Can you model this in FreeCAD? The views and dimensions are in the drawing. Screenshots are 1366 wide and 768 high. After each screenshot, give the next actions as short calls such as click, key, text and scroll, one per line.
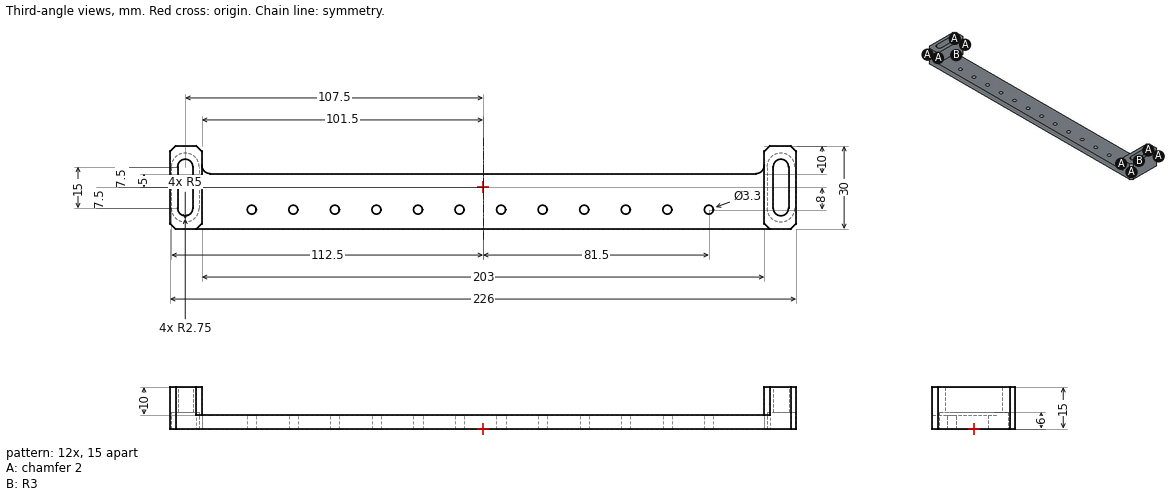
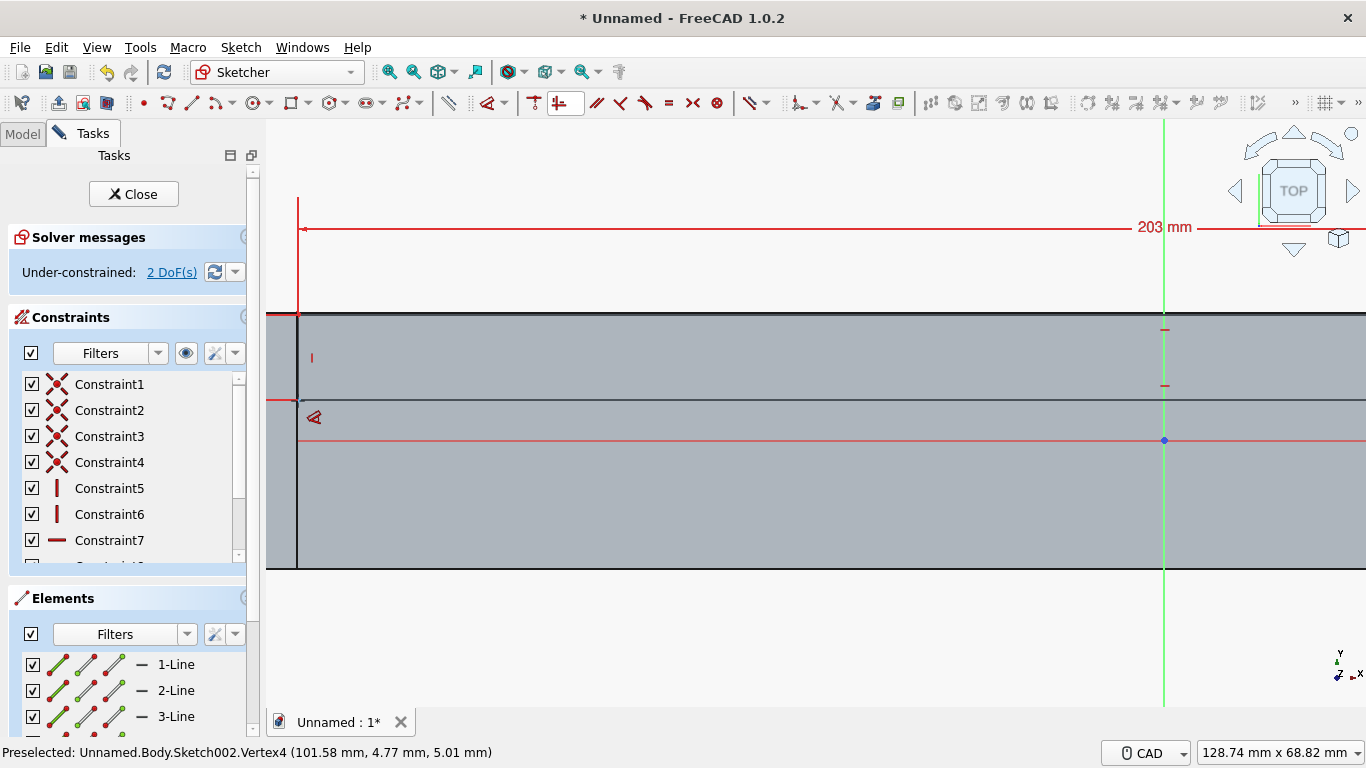
click(298, 400)
click(1198, 420)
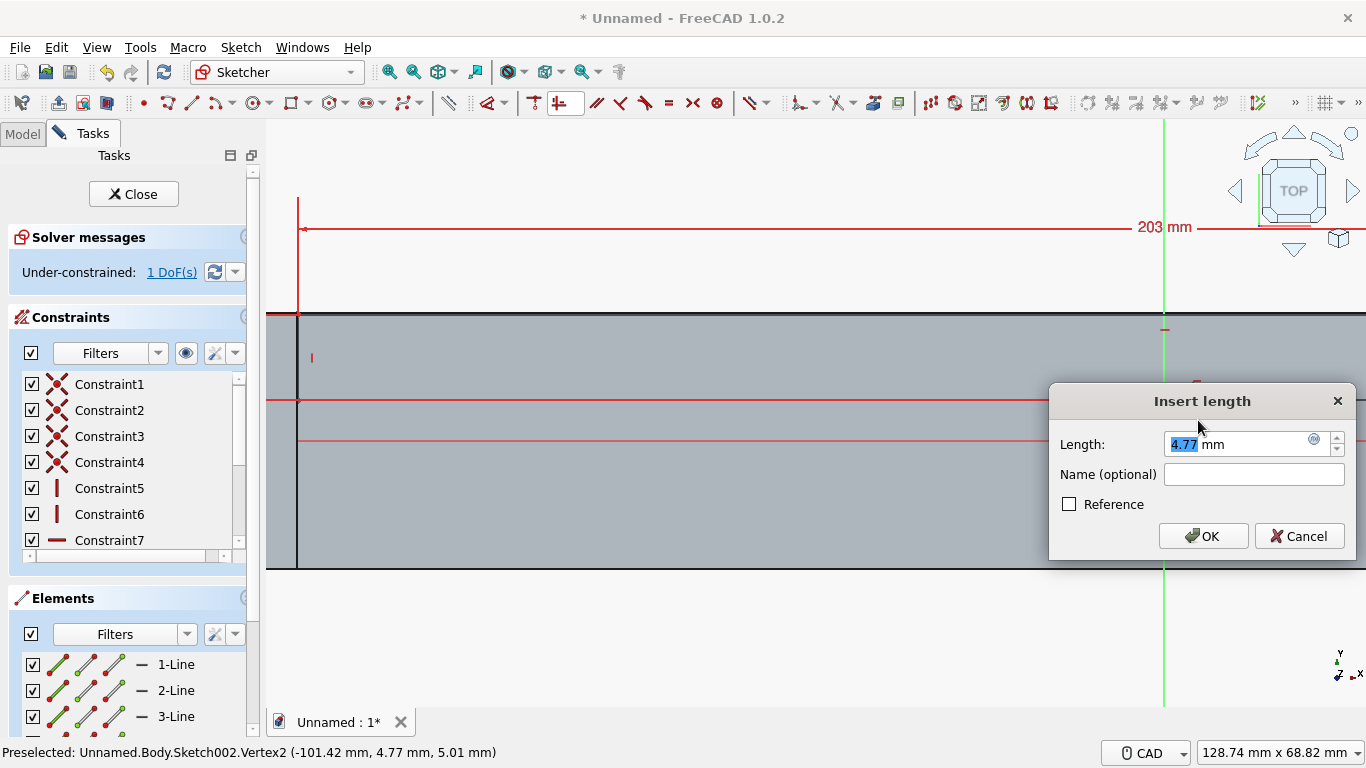
text(5)
key(Return)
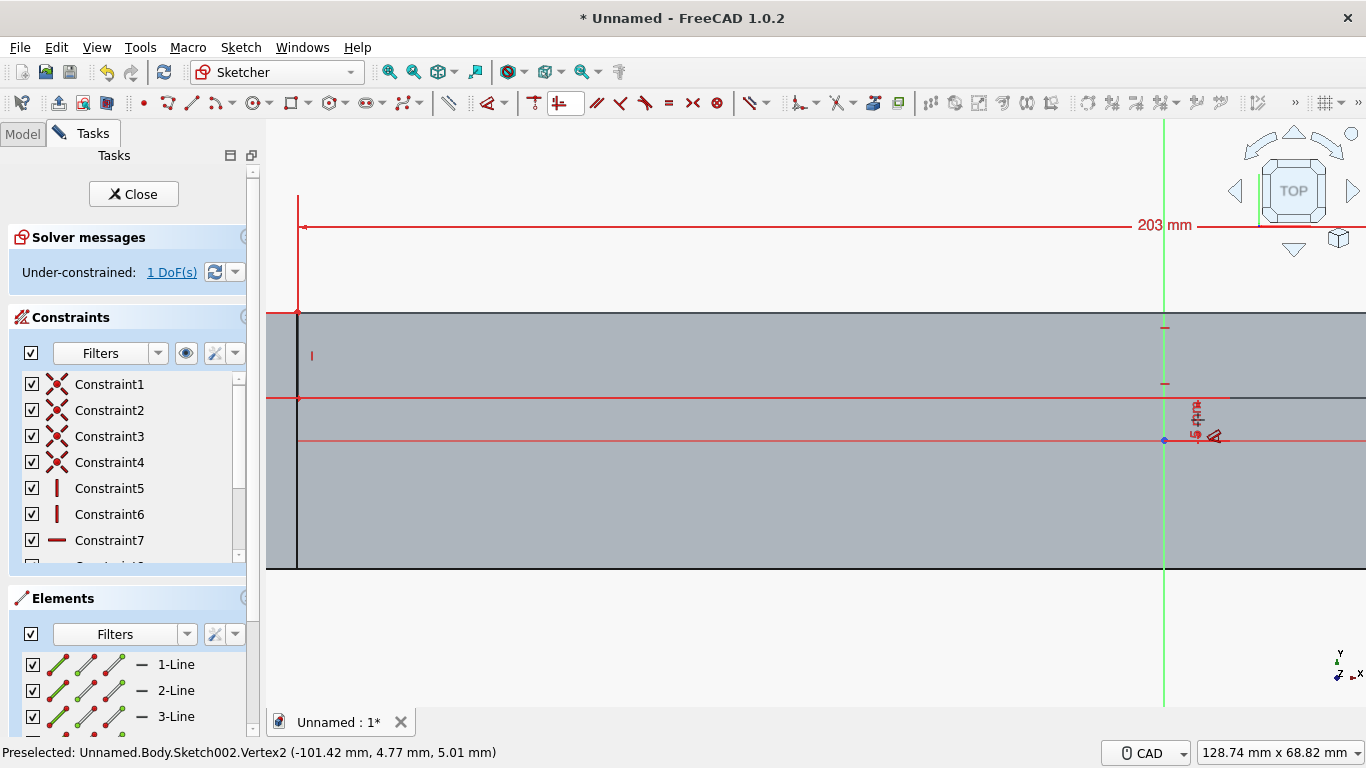
click(298, 313)
click(731, 475)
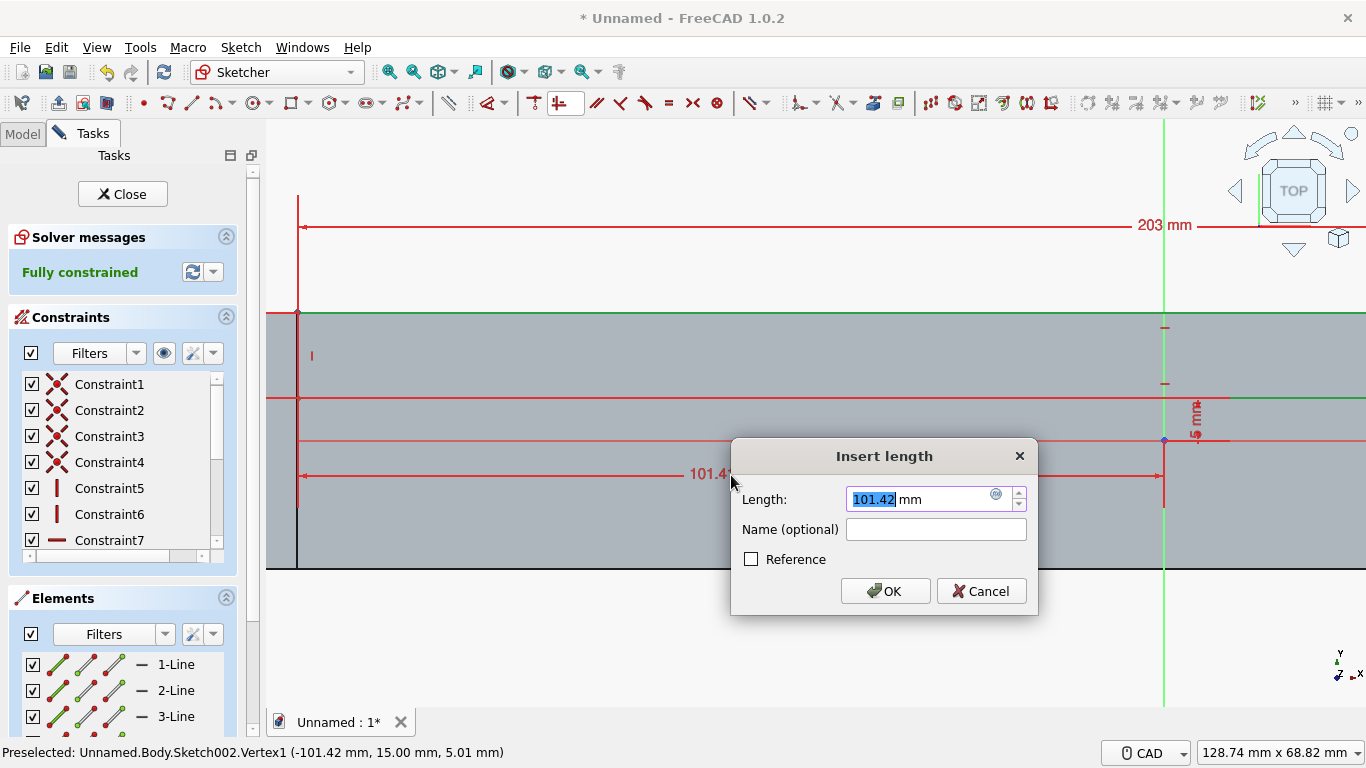
text(101.5)
key(Return)
key(Escape)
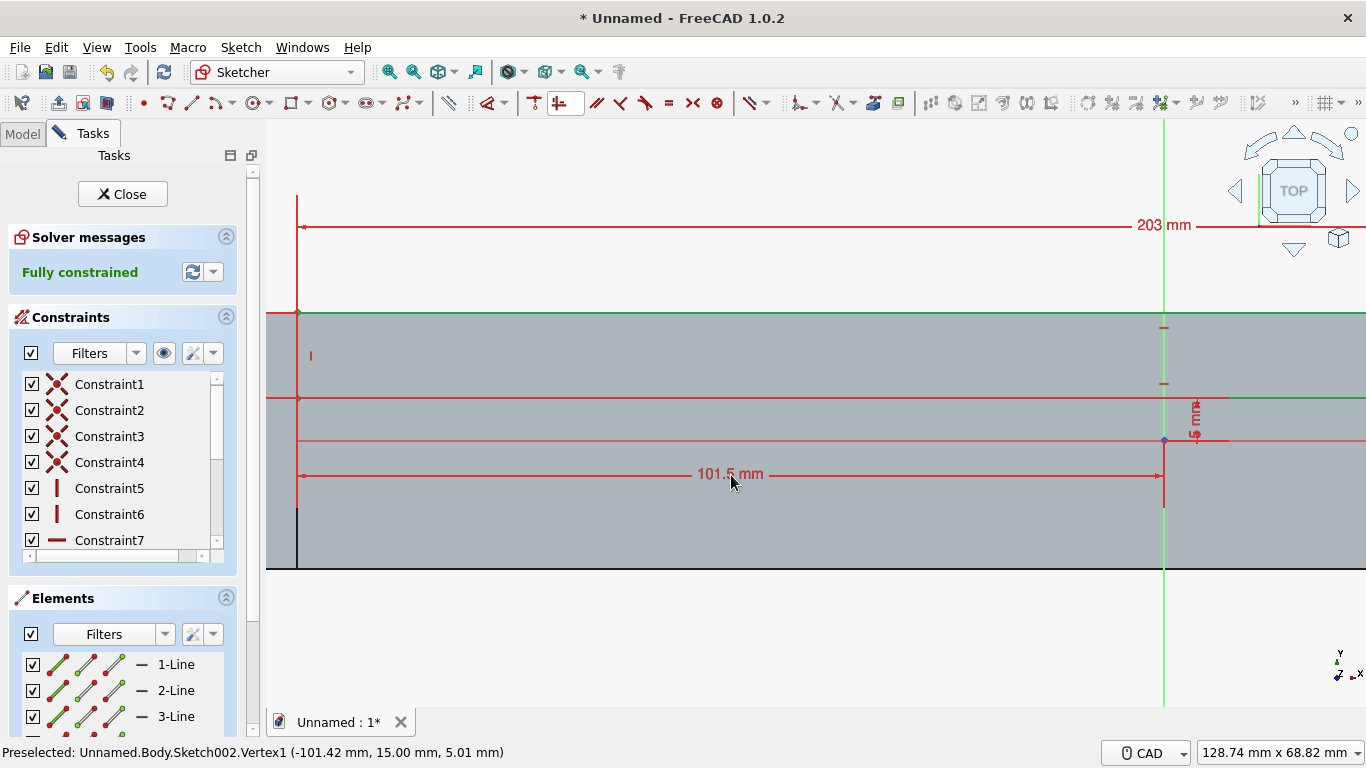
click(123, 194)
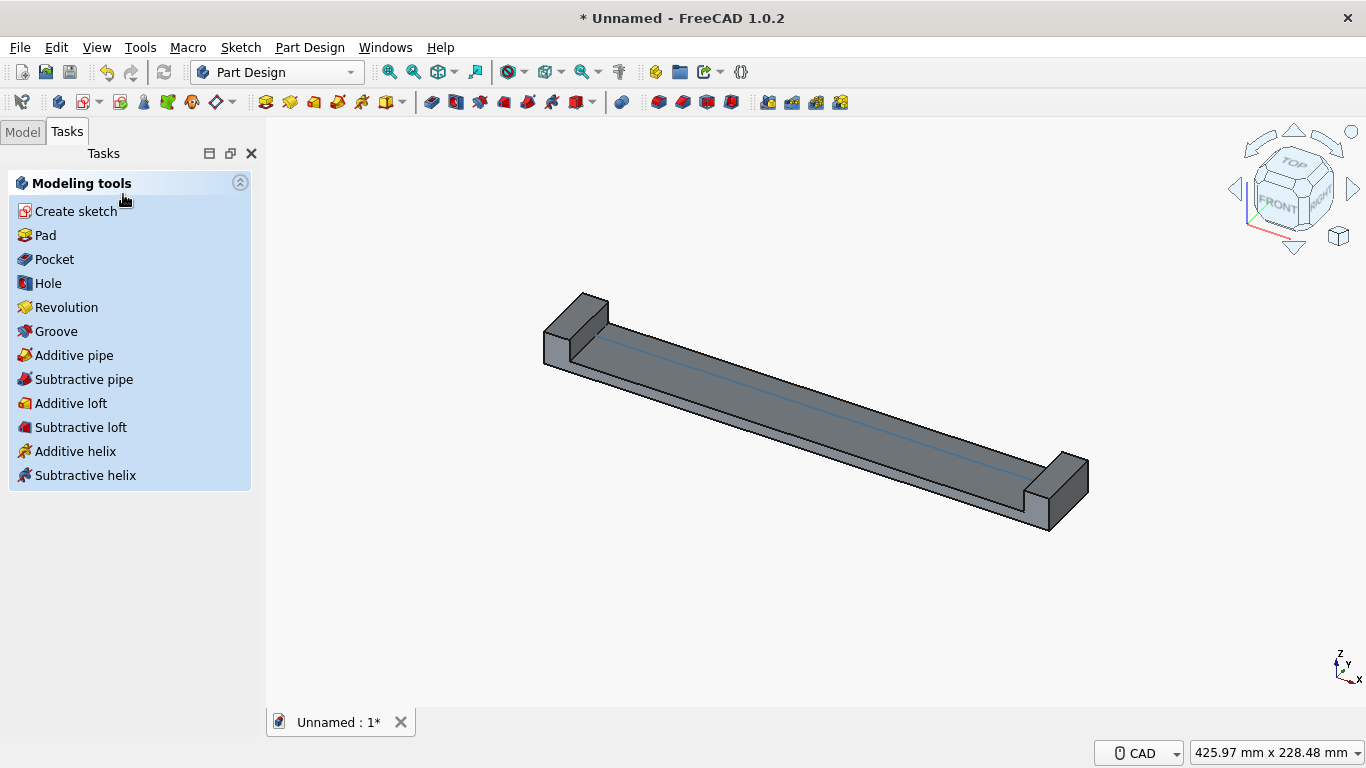
click(432, 102)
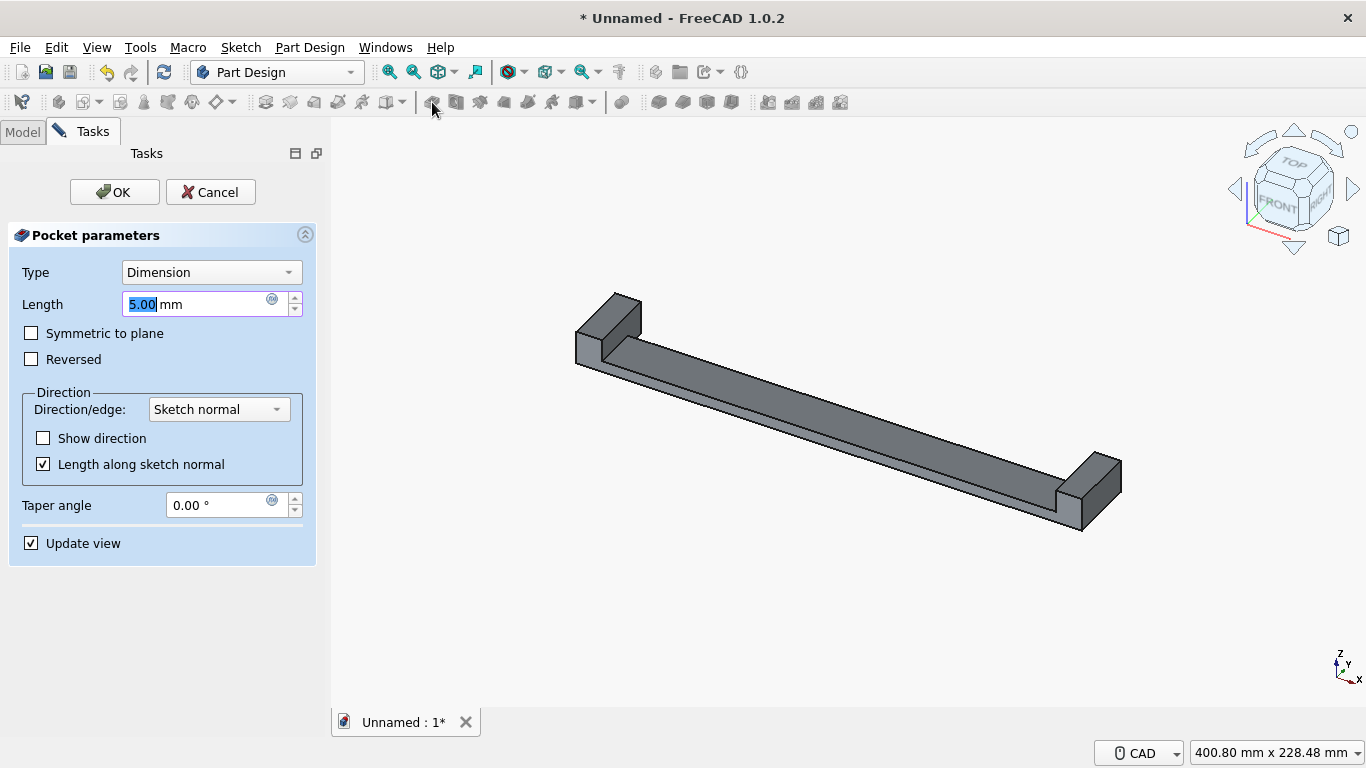
click(212, 272)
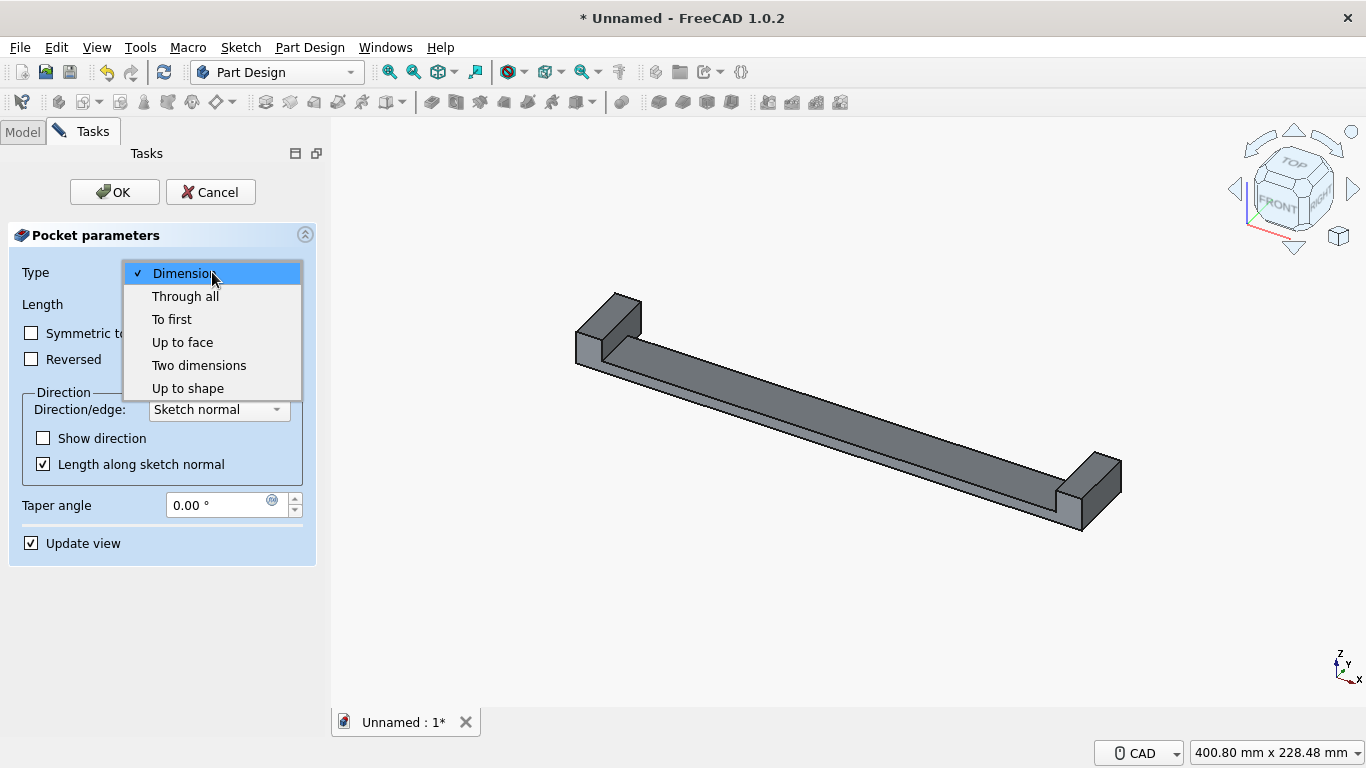
click(212, 296)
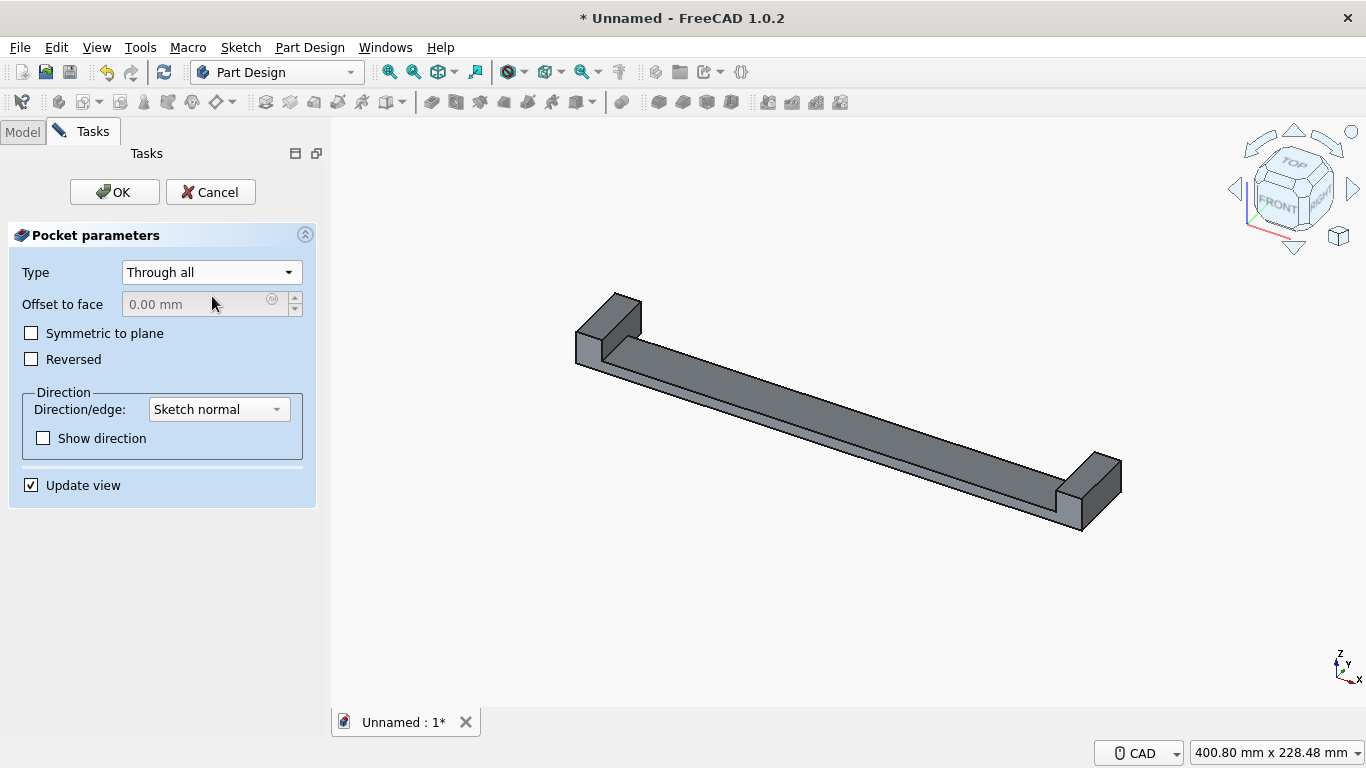
click(115, 192)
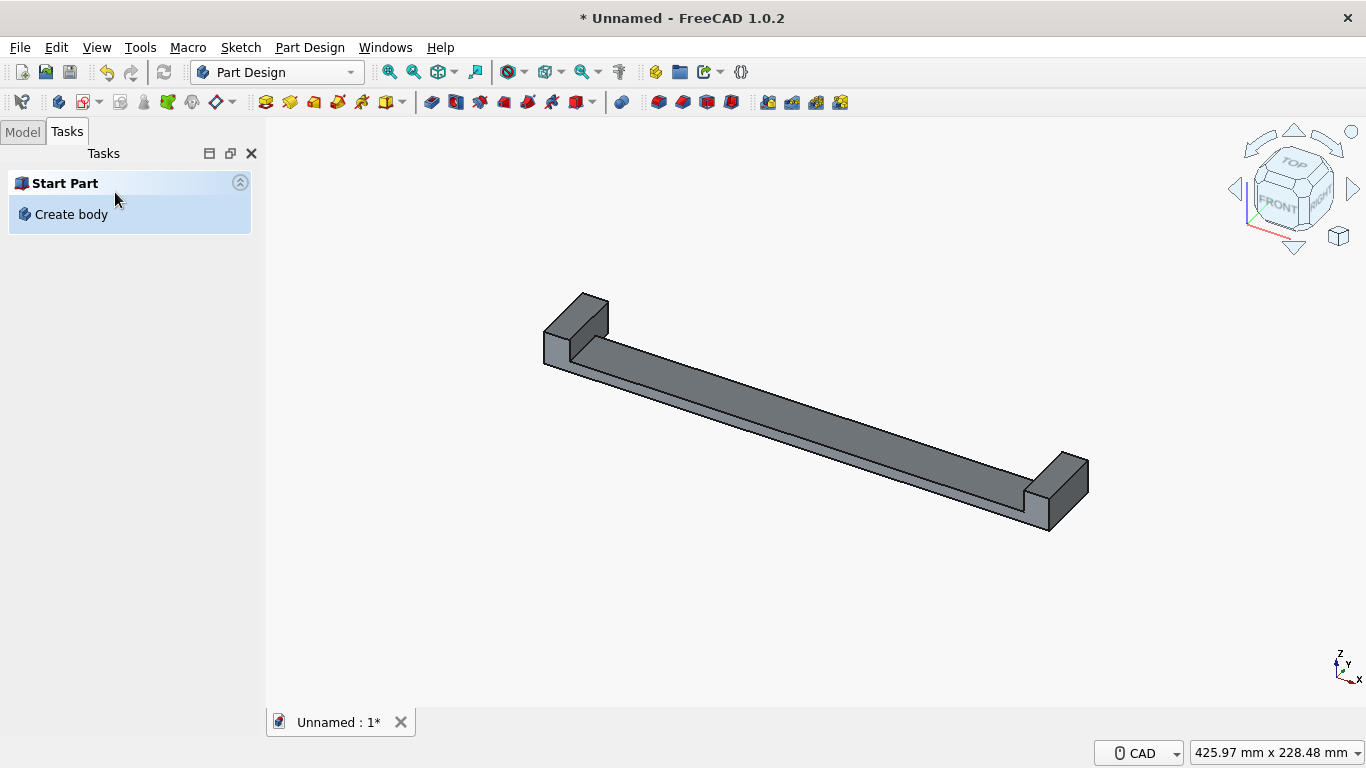
key(5)